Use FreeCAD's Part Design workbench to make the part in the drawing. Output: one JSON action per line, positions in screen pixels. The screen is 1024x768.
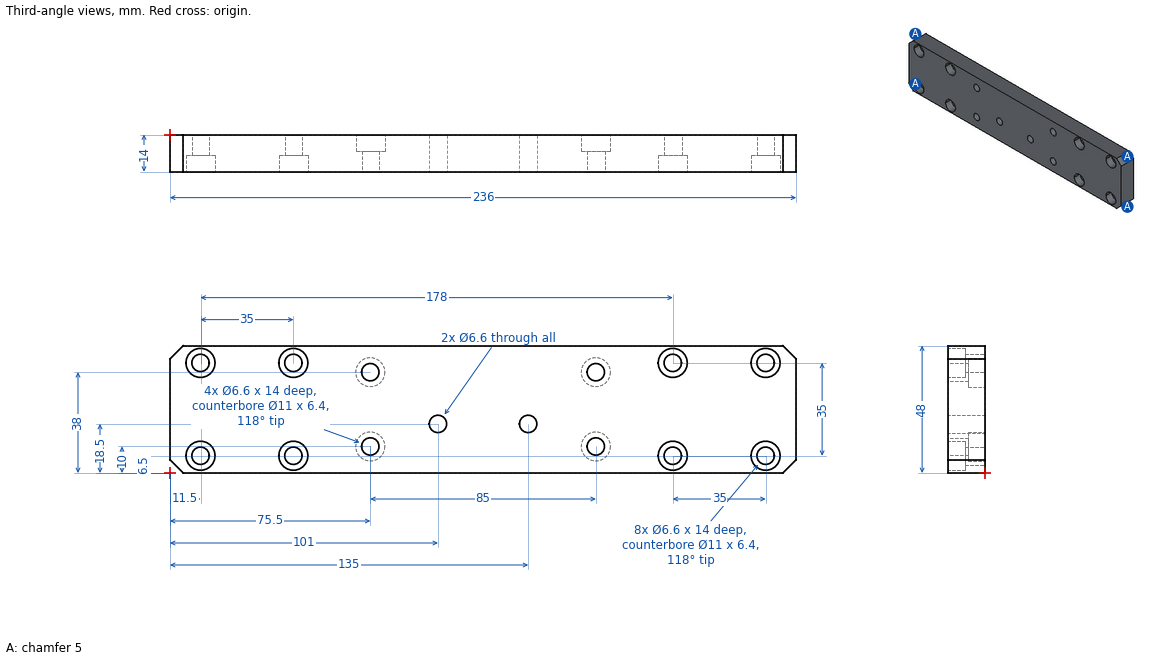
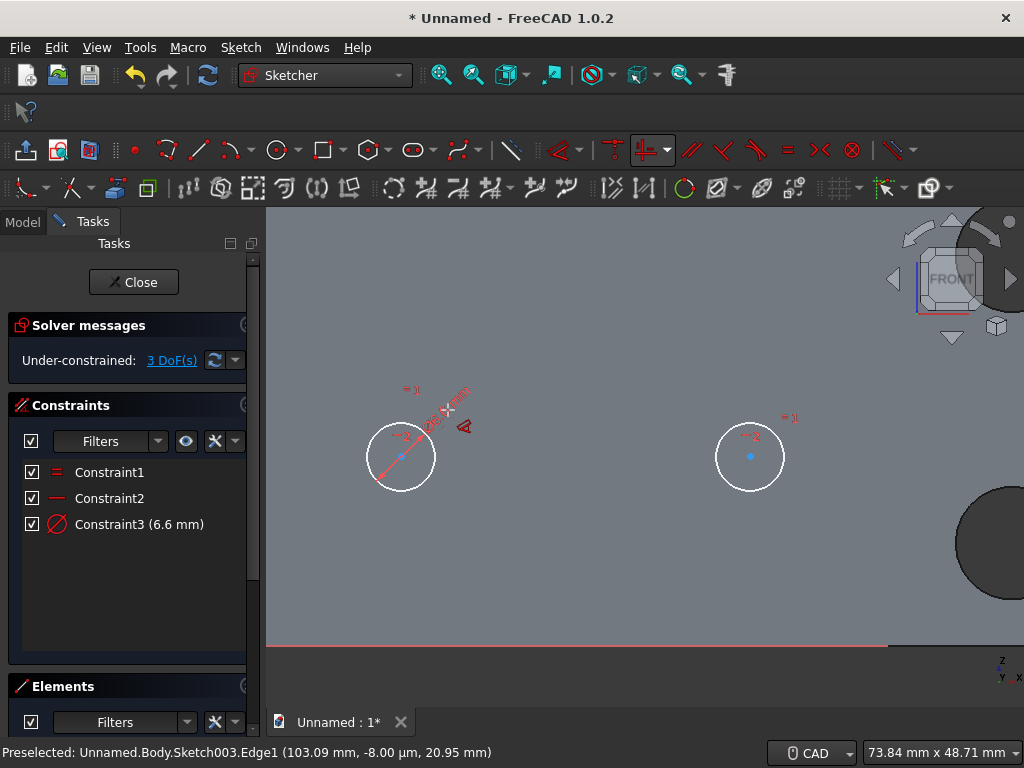
{"action": "left_click", "coordinate": [401, 457]}
{"action": "left_click", "coordinate": [348, 423]}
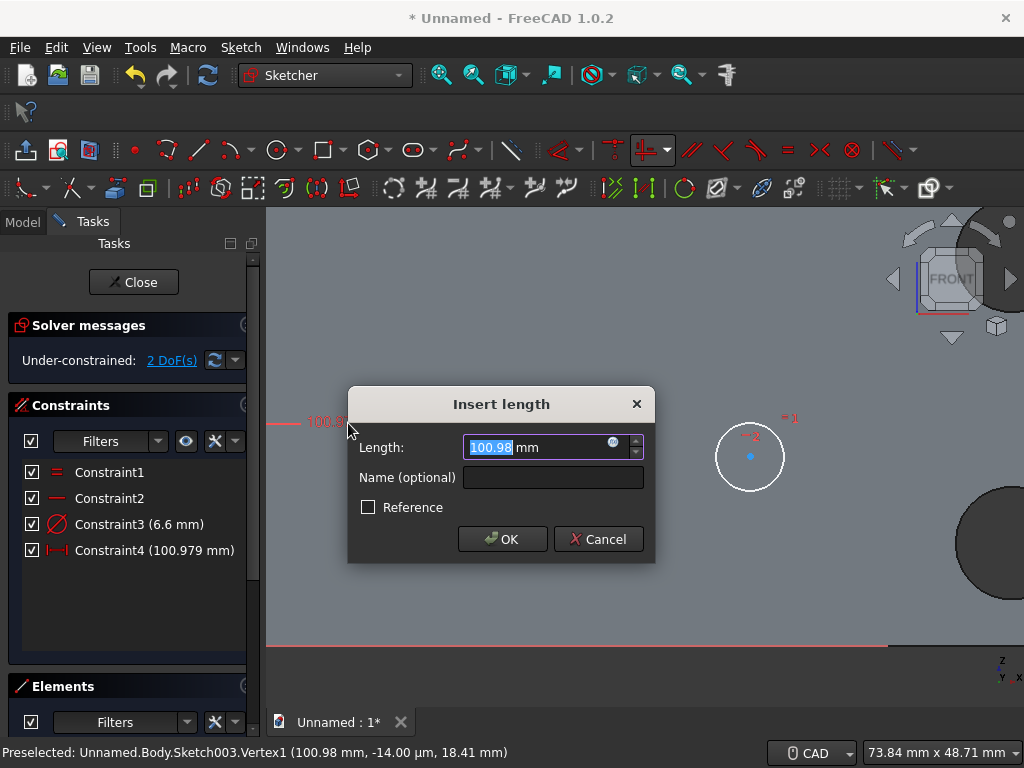
{"action": "type", "text": "101"}
{"action": "key", "text": "Return"}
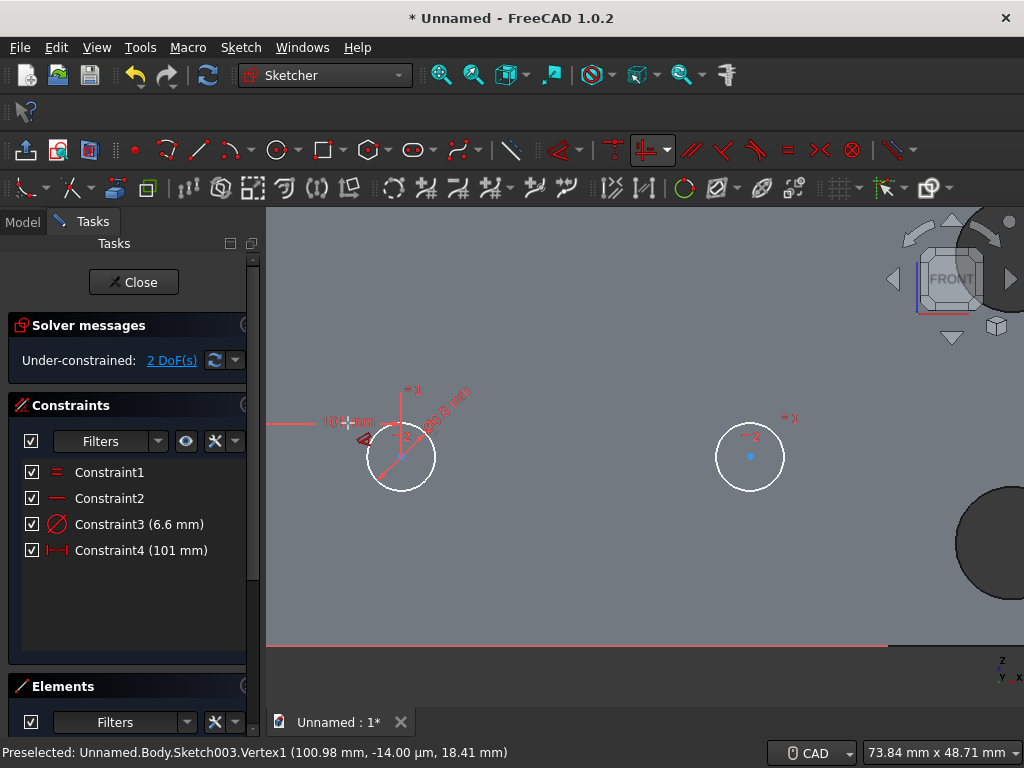
{"action": "left_click", "coordinate": [750, 457]}
{"action": "left_click", "coordinate": [522, 423]}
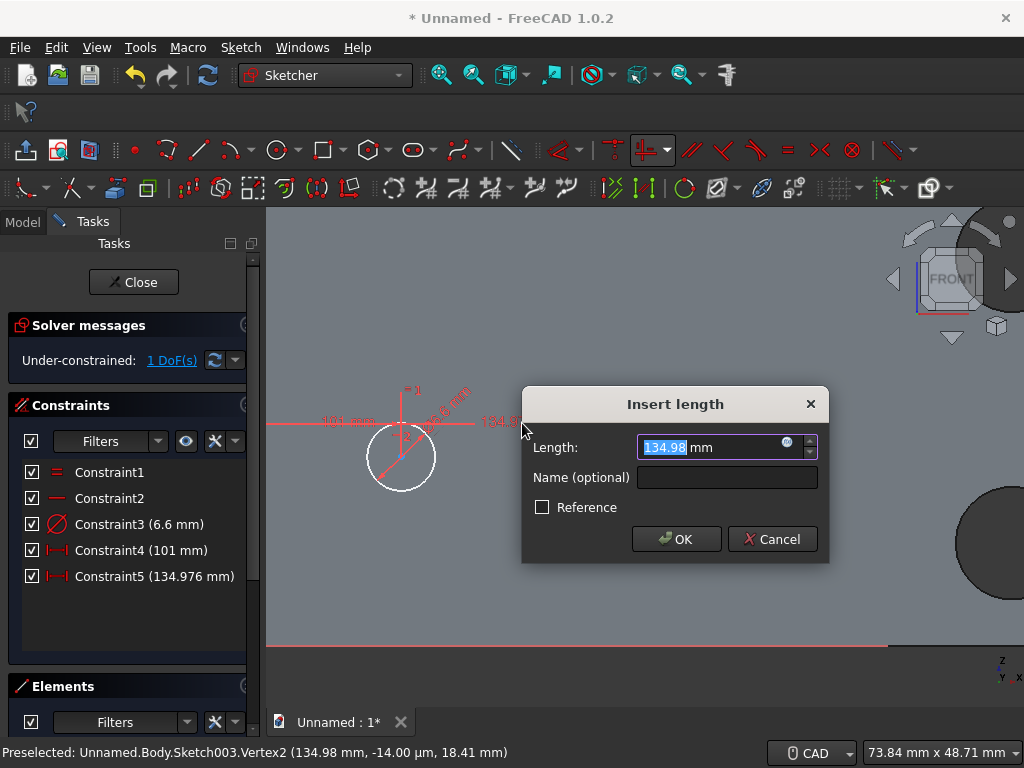
{"action": "type", "text": "135"}
{"action": "key", "text": "Return"}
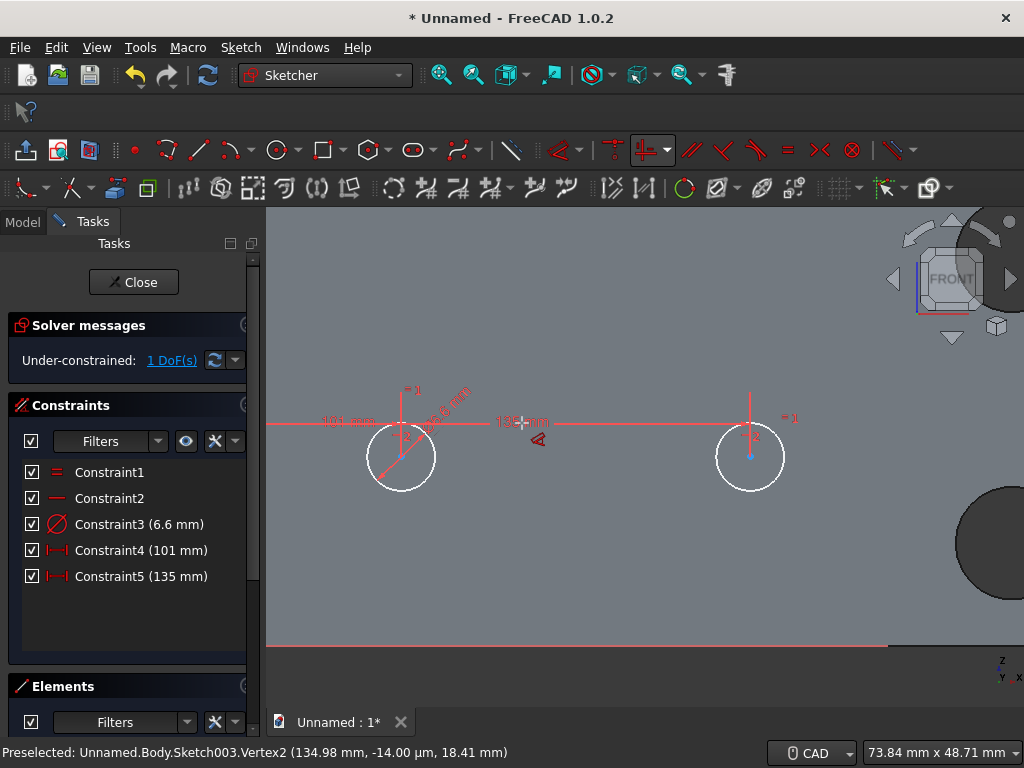
{"action": "left_click", "coordinate": [401, 457]}
{"action": "left_click", "coordinate": [435, 551]}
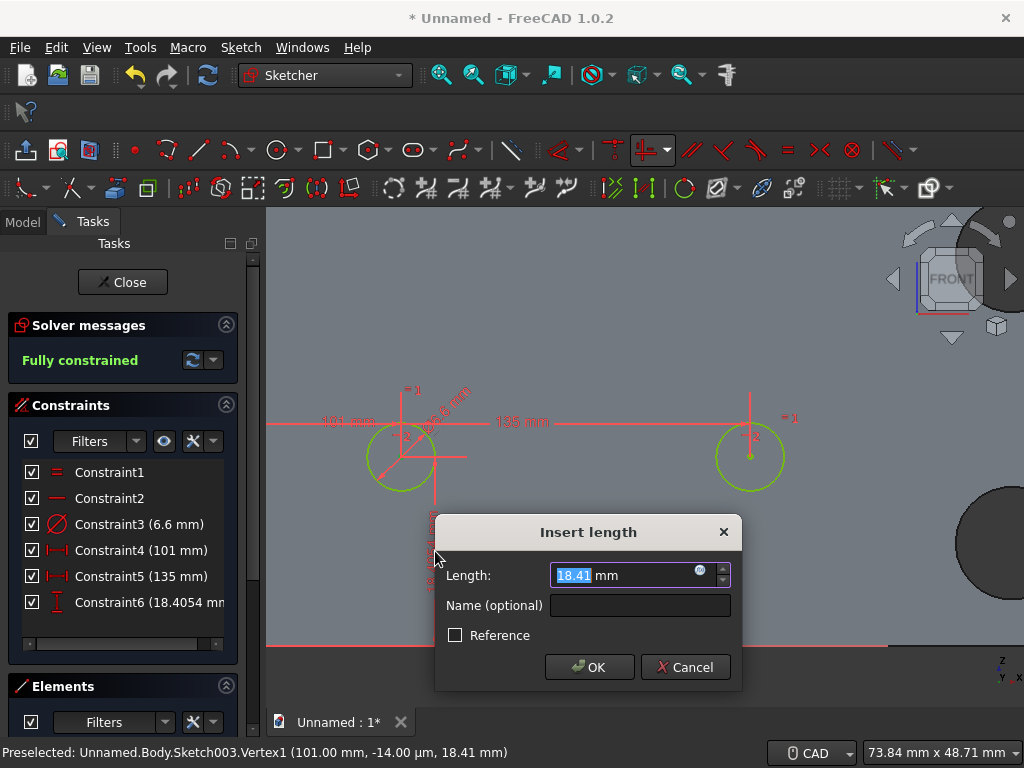
{"action": "type", "text": "18.5"}
{"action": "key", "text": "Return"}
{"action": "key", "text": "Escape"}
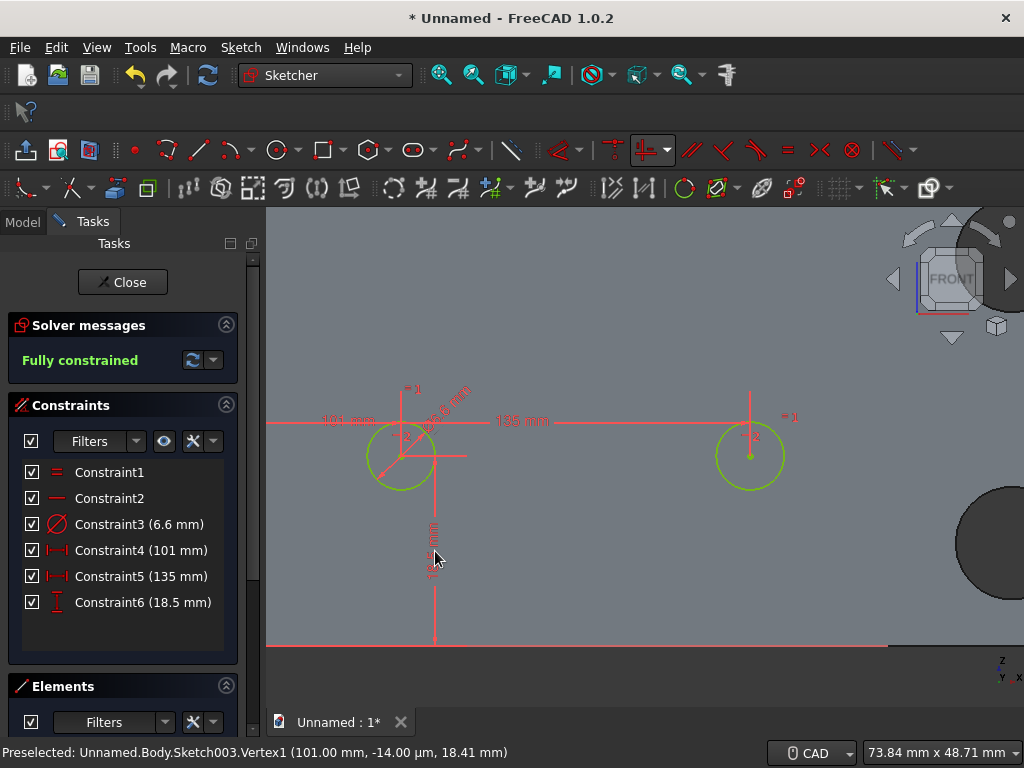
{"action": "left_click", "coordinate": [123, 282]}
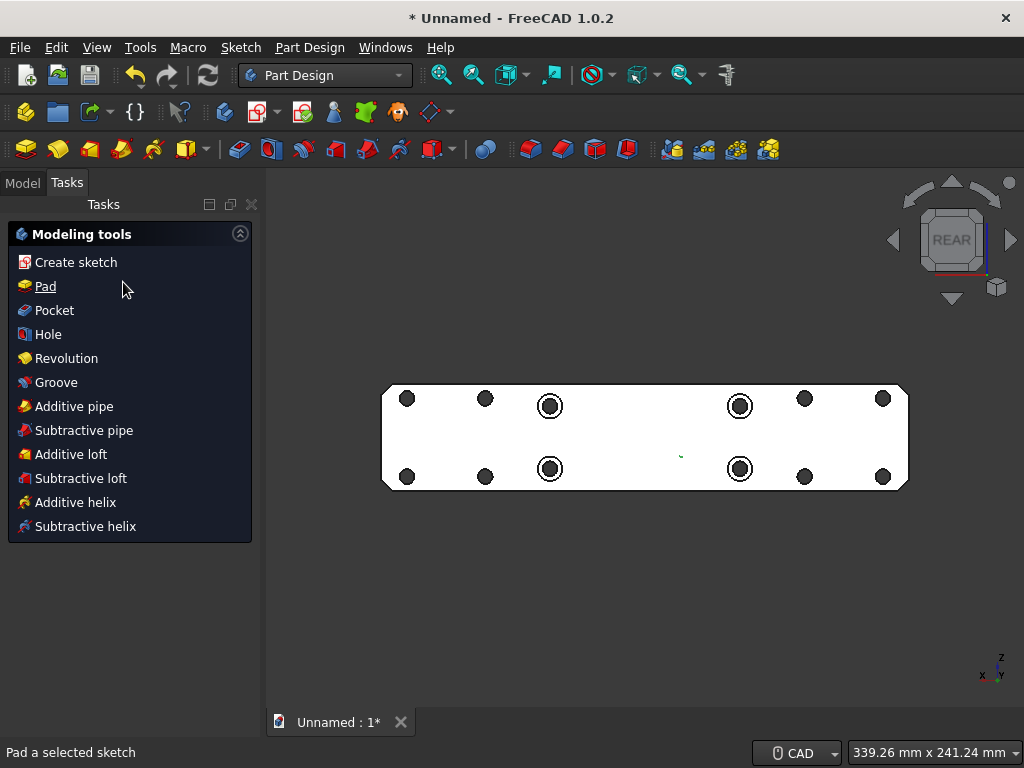
{"action": "left_click", "coordinate": [272, 150]}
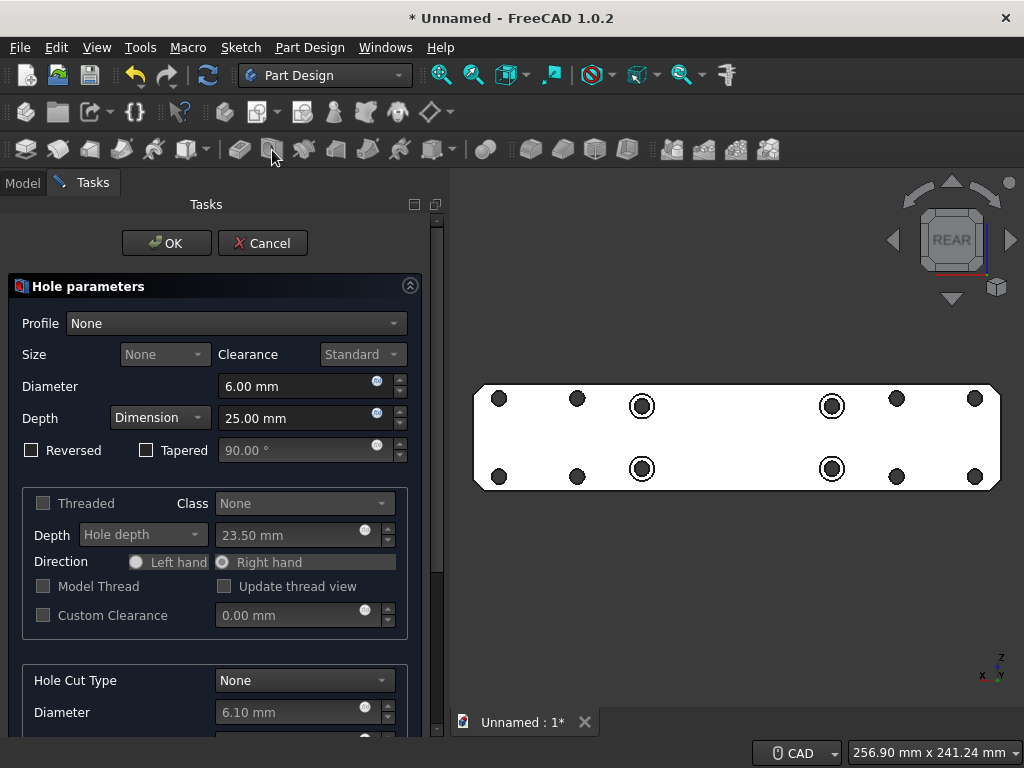
{"action": "triple_click", "coordinate": [305, 386]}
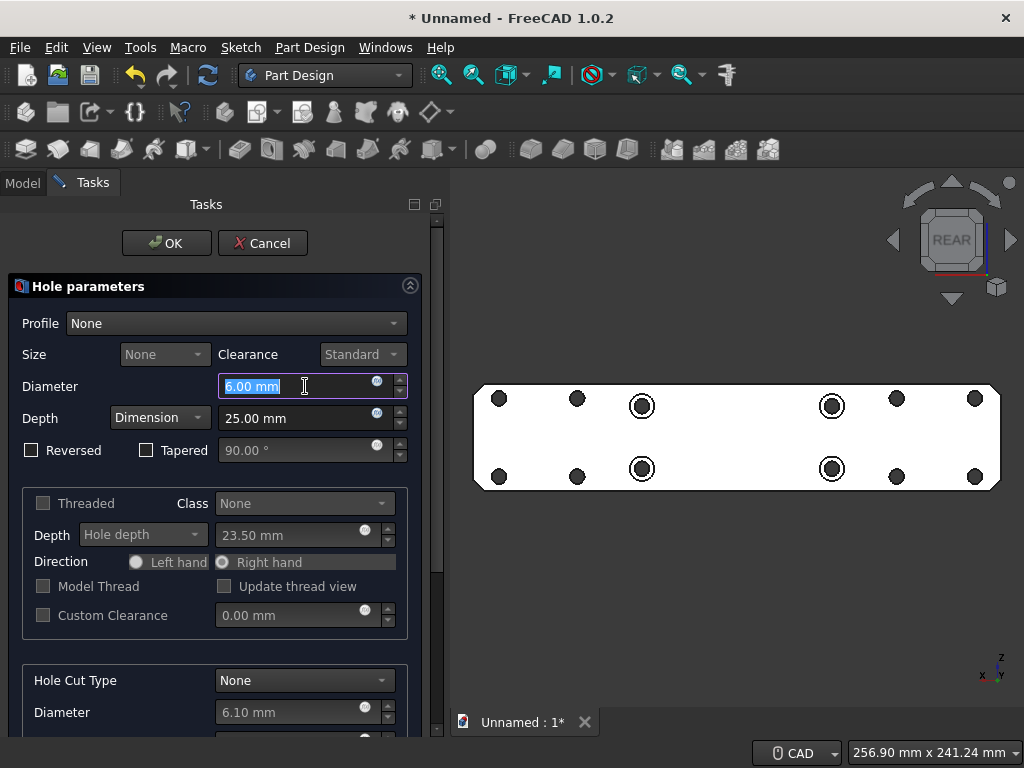
{"action": "type", "text": "6.6"}
{"action": "key", "text": "Tab"}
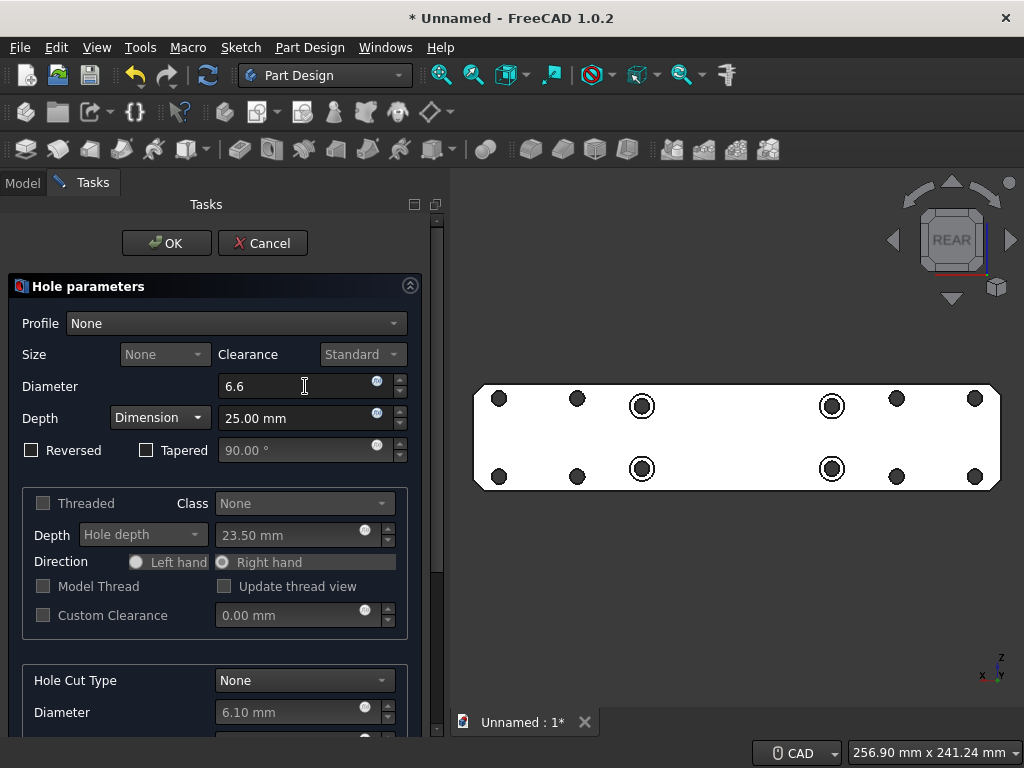
{"action": "left_click", "coordinate": [161, 418]}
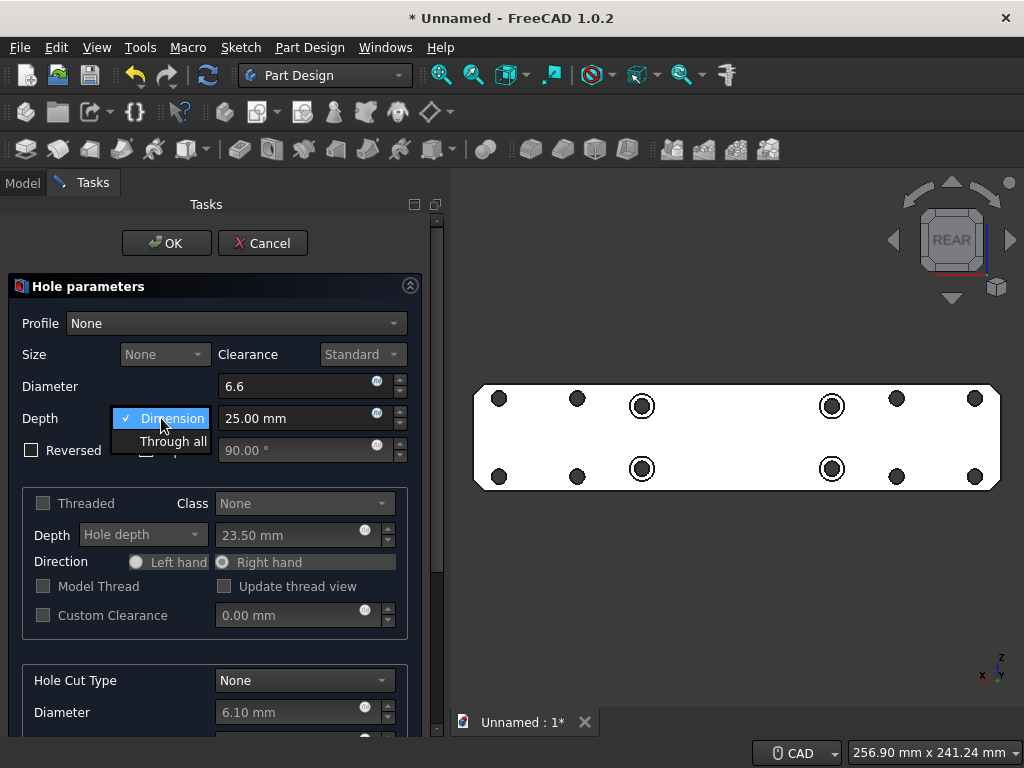
{"action": "left_click", "coordinate": [160, 442]}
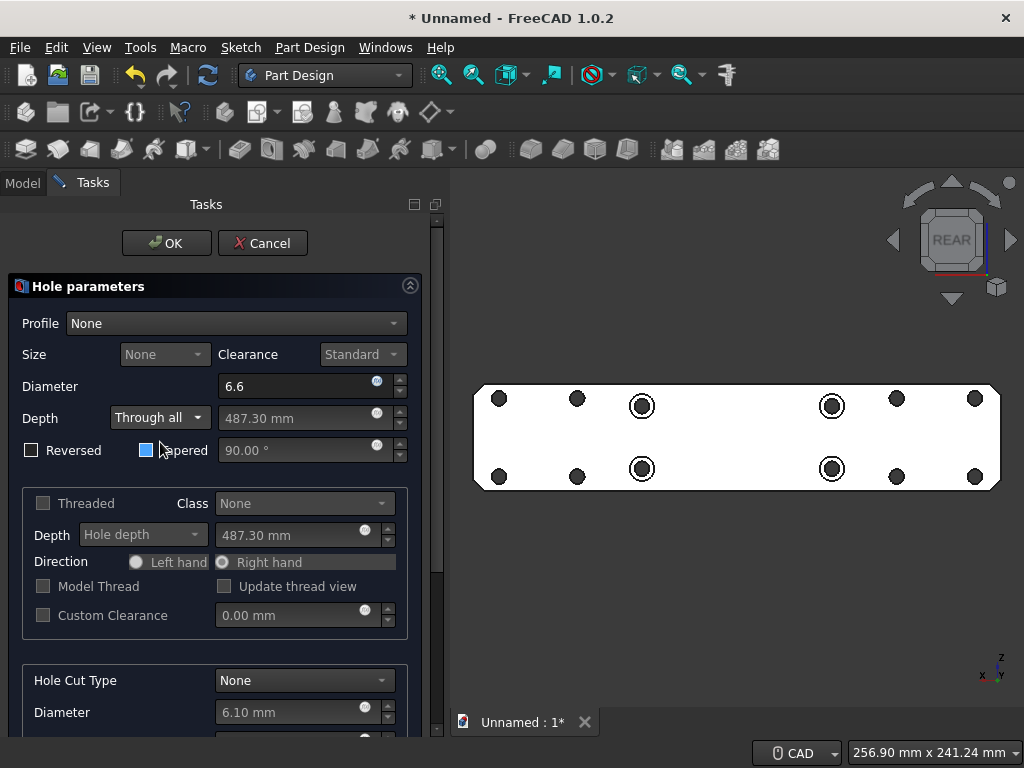
{"action": "left_click", "coordinate": [30, 450]}